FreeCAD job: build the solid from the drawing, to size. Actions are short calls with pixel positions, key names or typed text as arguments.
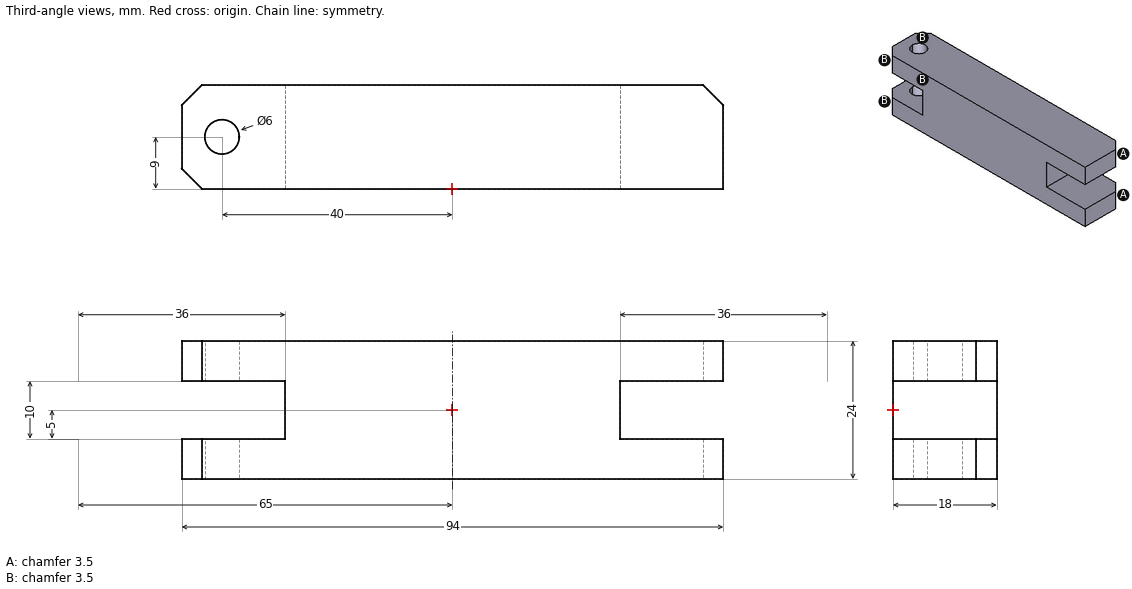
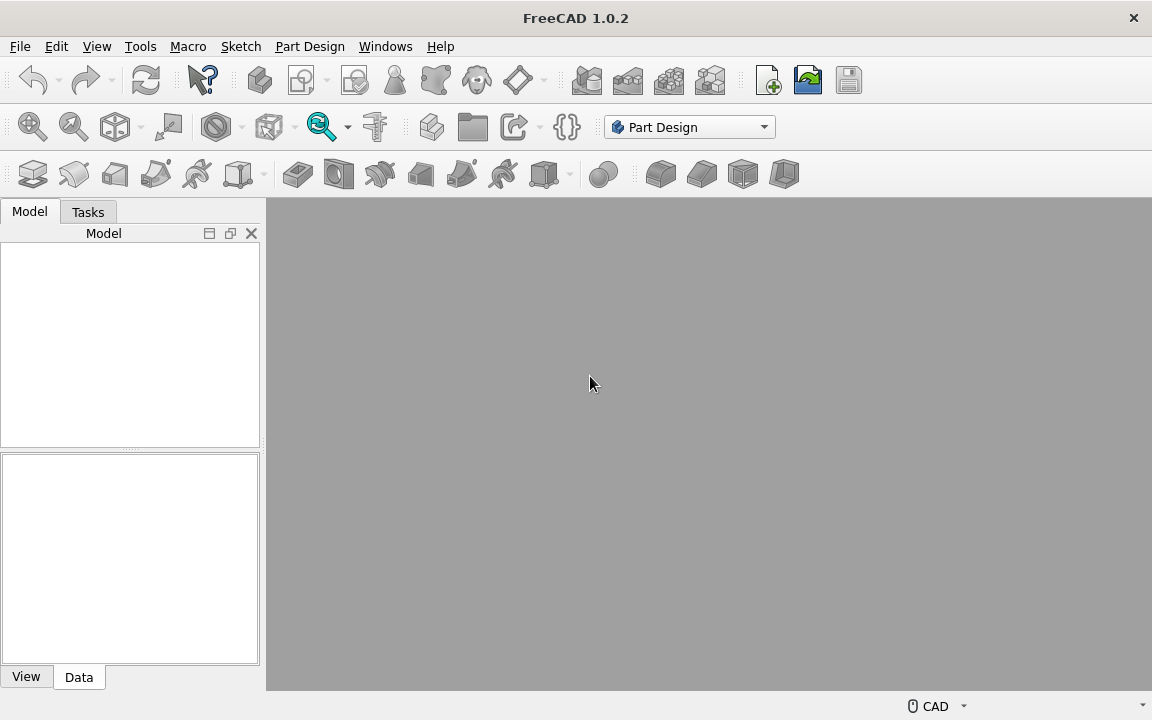
key(ctrl+n)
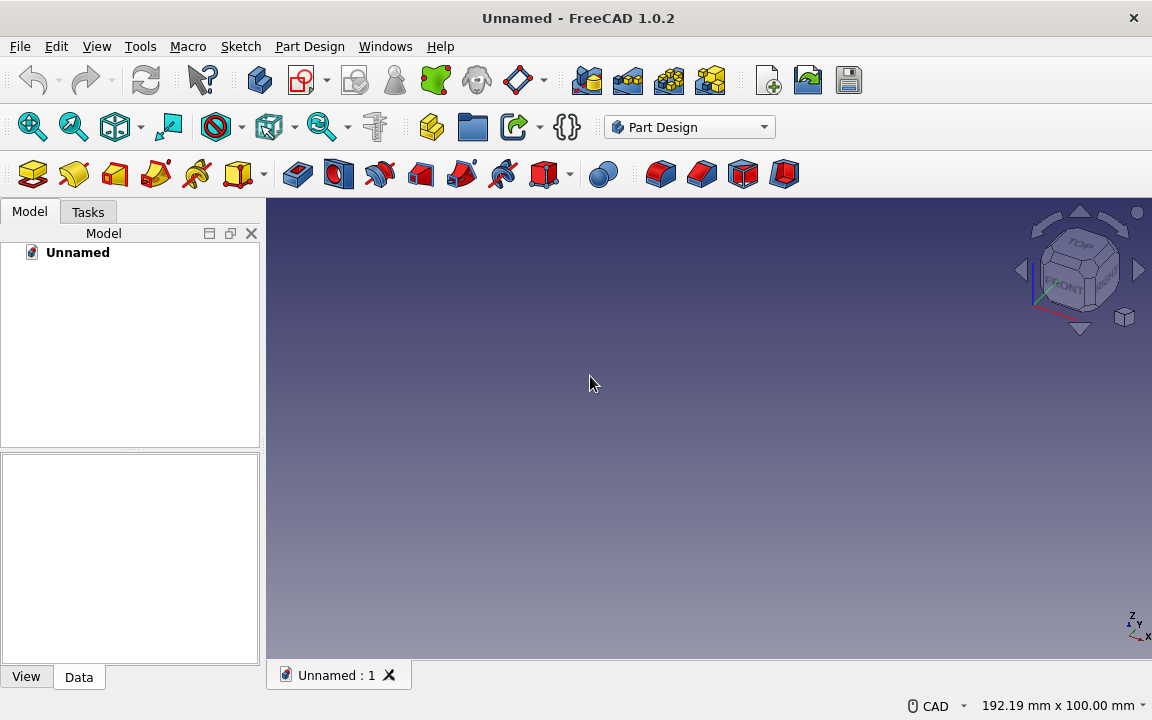
click(300, 80)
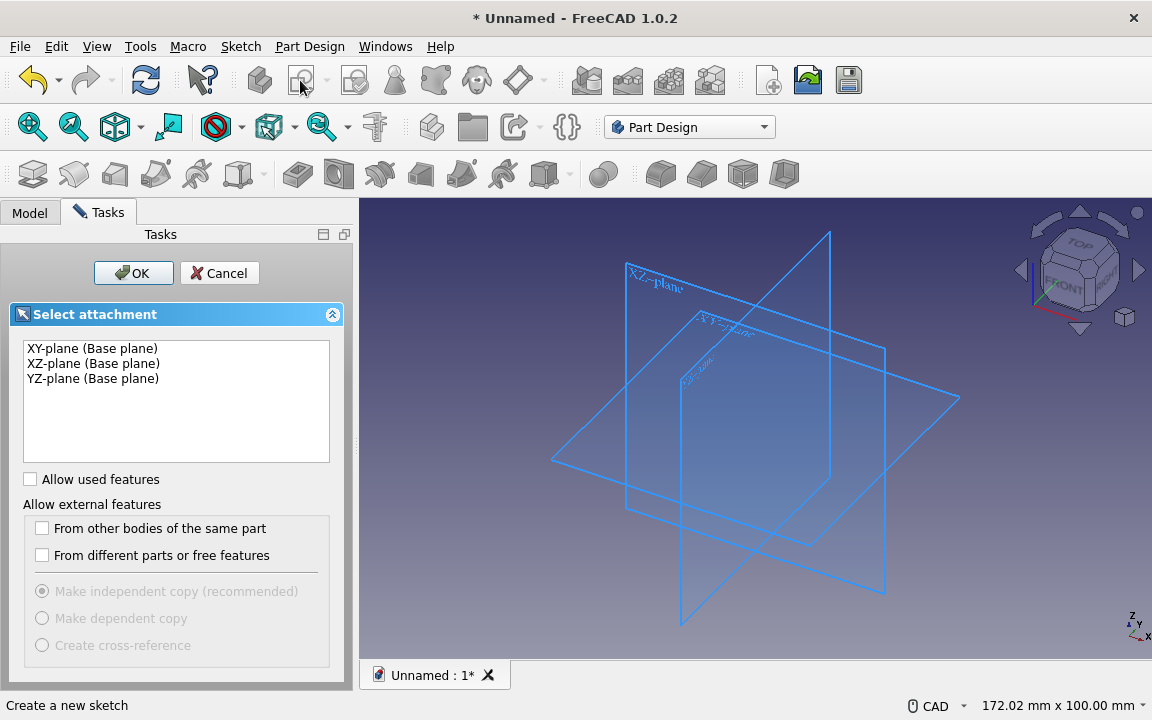
click(84, 364)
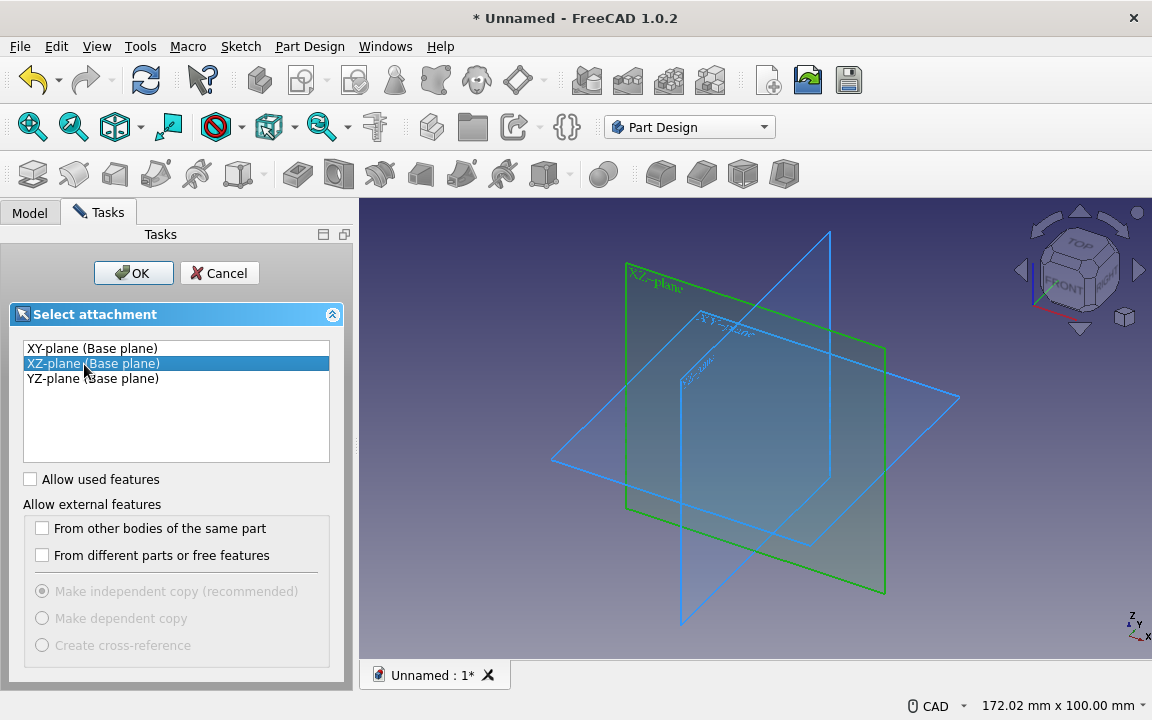
click(134, 273)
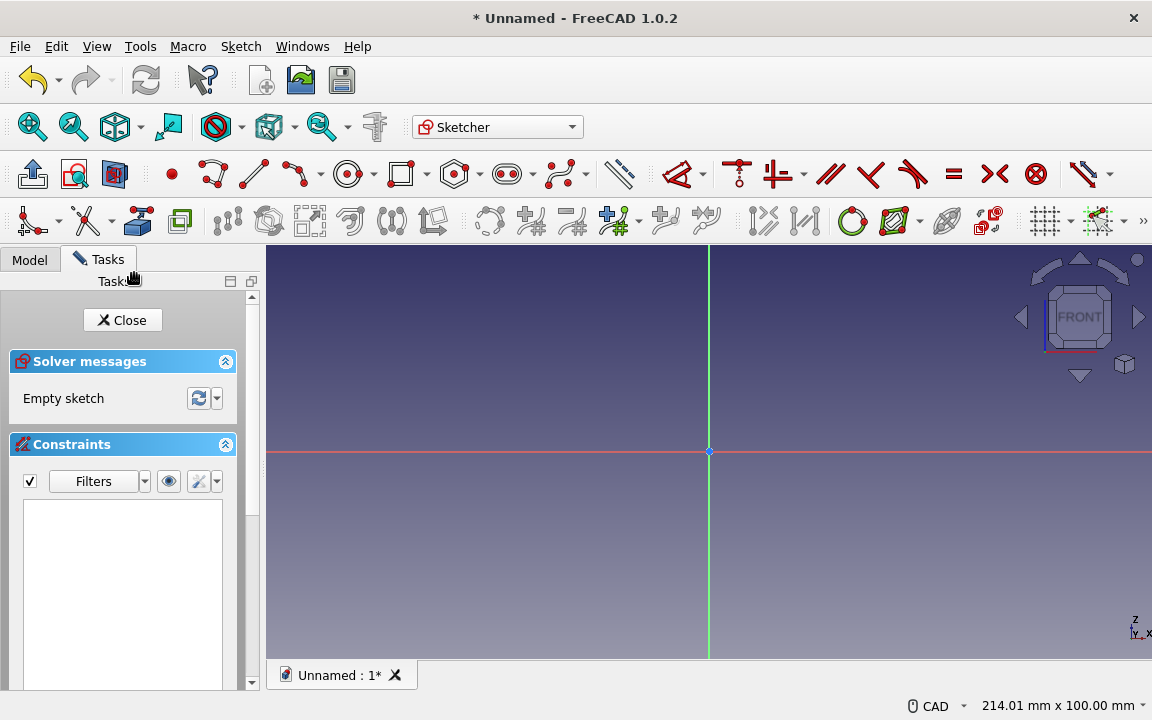
key(g)
key(v)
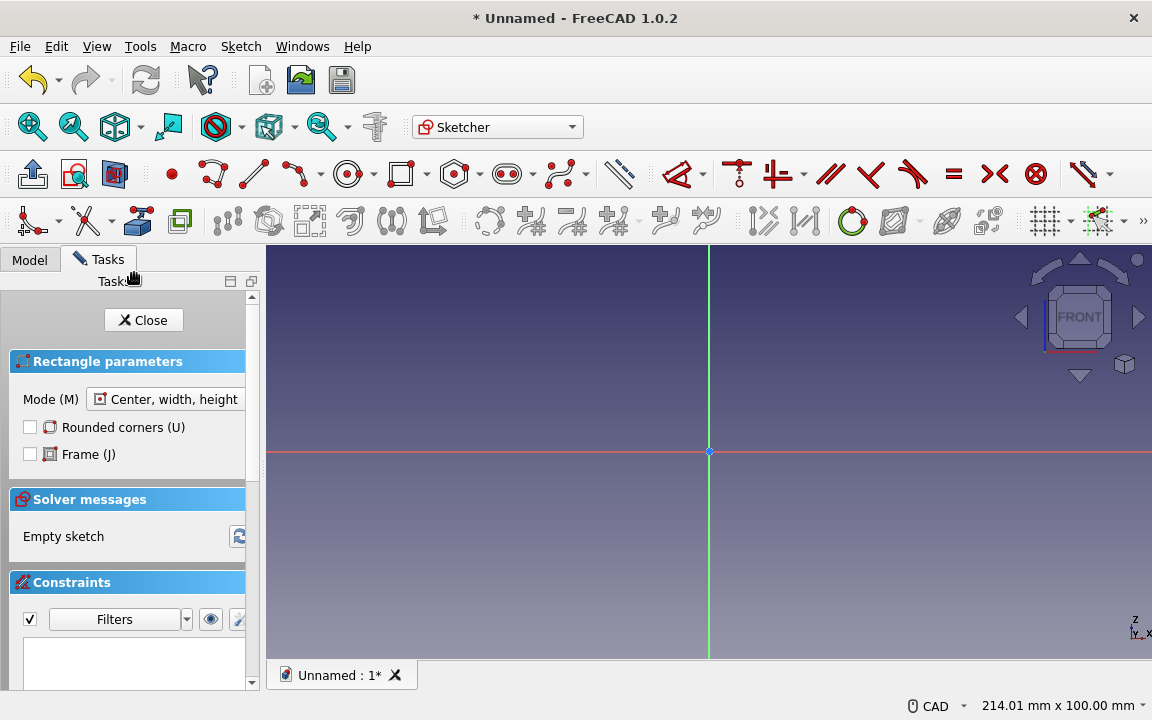
click(709, 452)
move(904, 402)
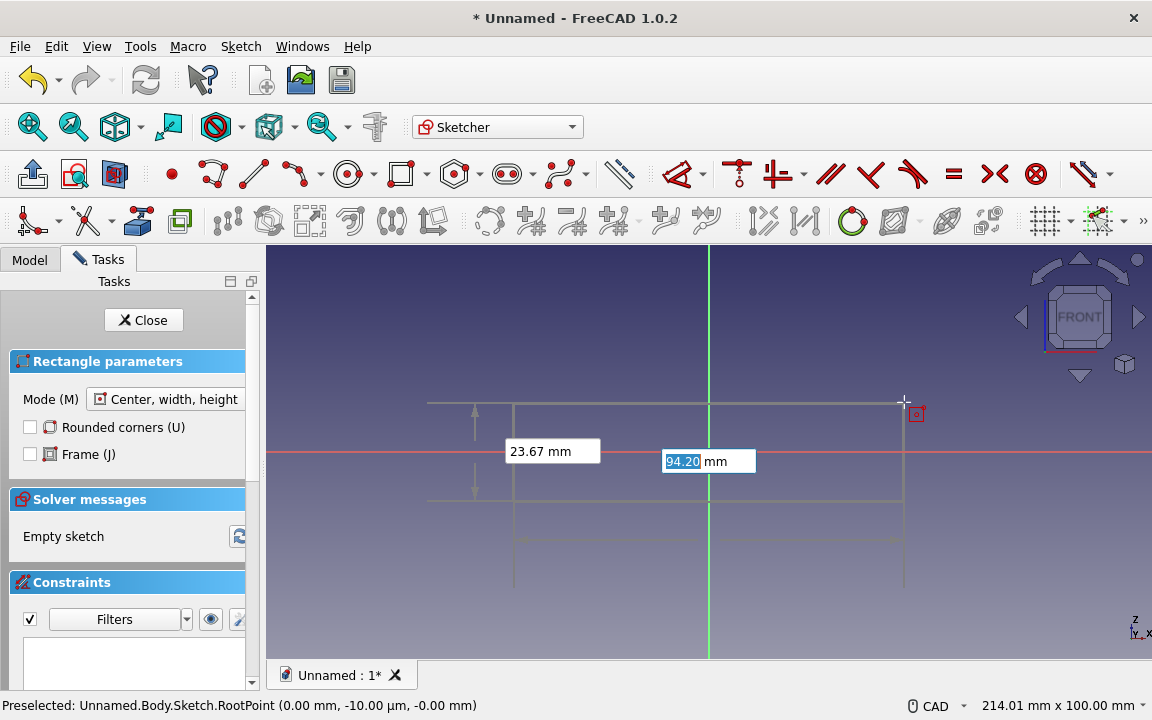
text(94)
key(Tab)
text(24)
key(Return)
key(Escape)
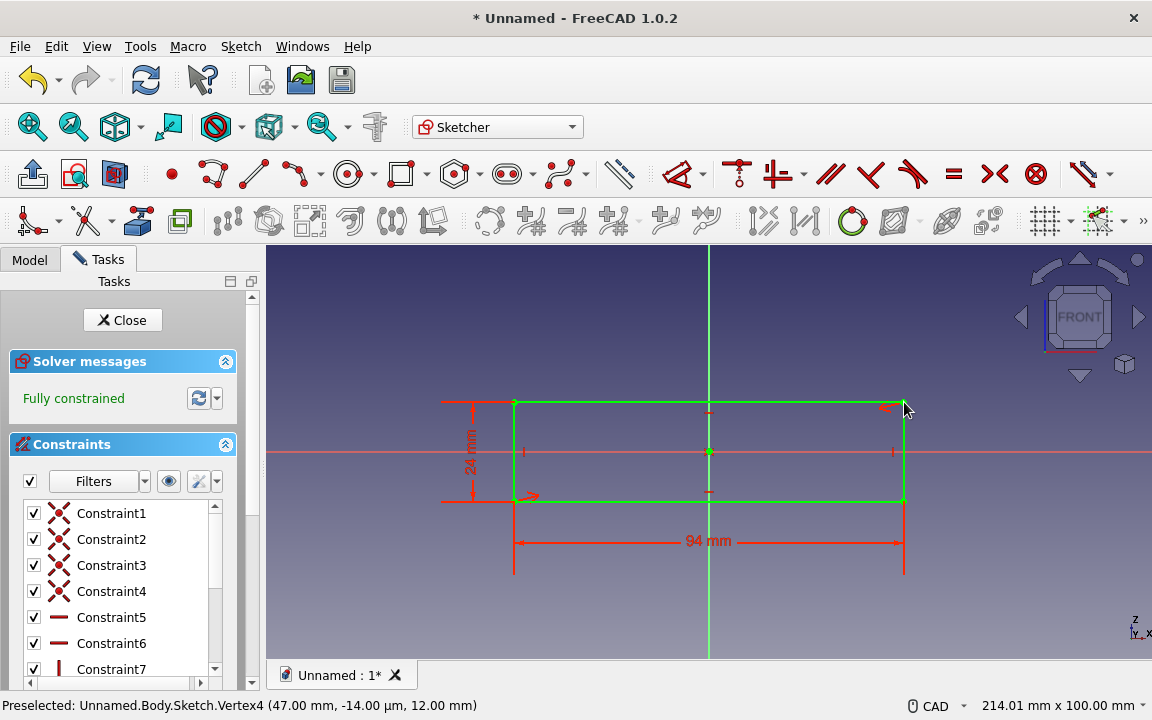
click(123, 320)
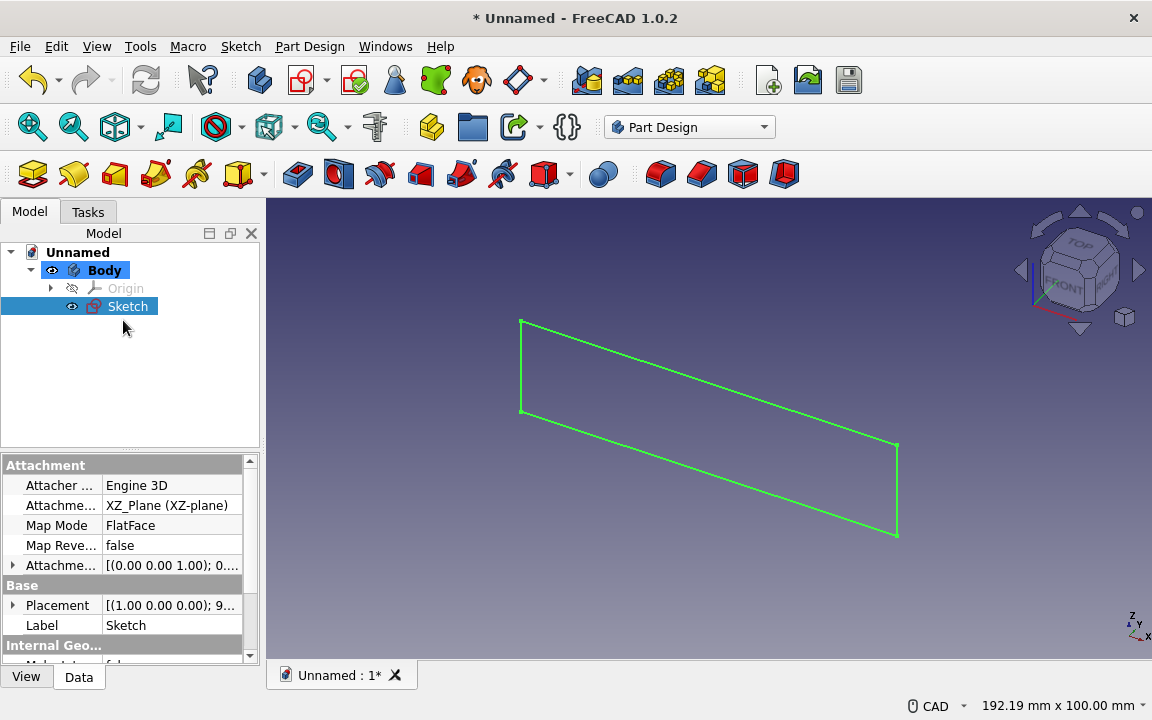
click(33, 174)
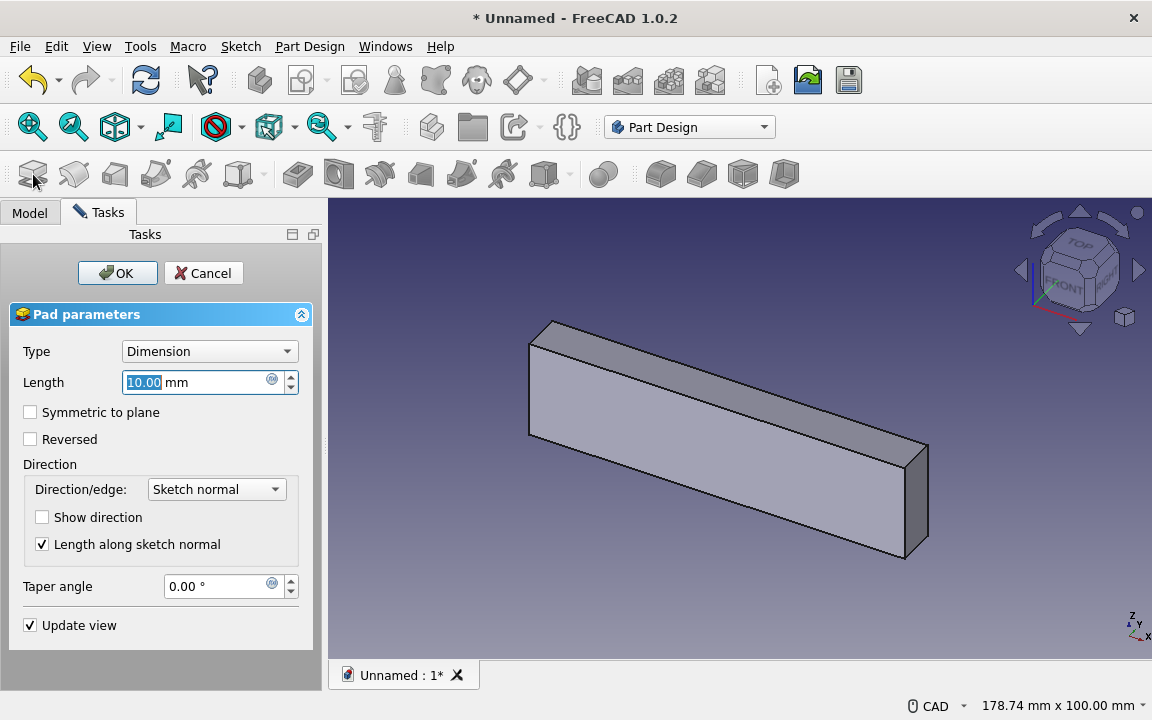
text(18)
key(Tab)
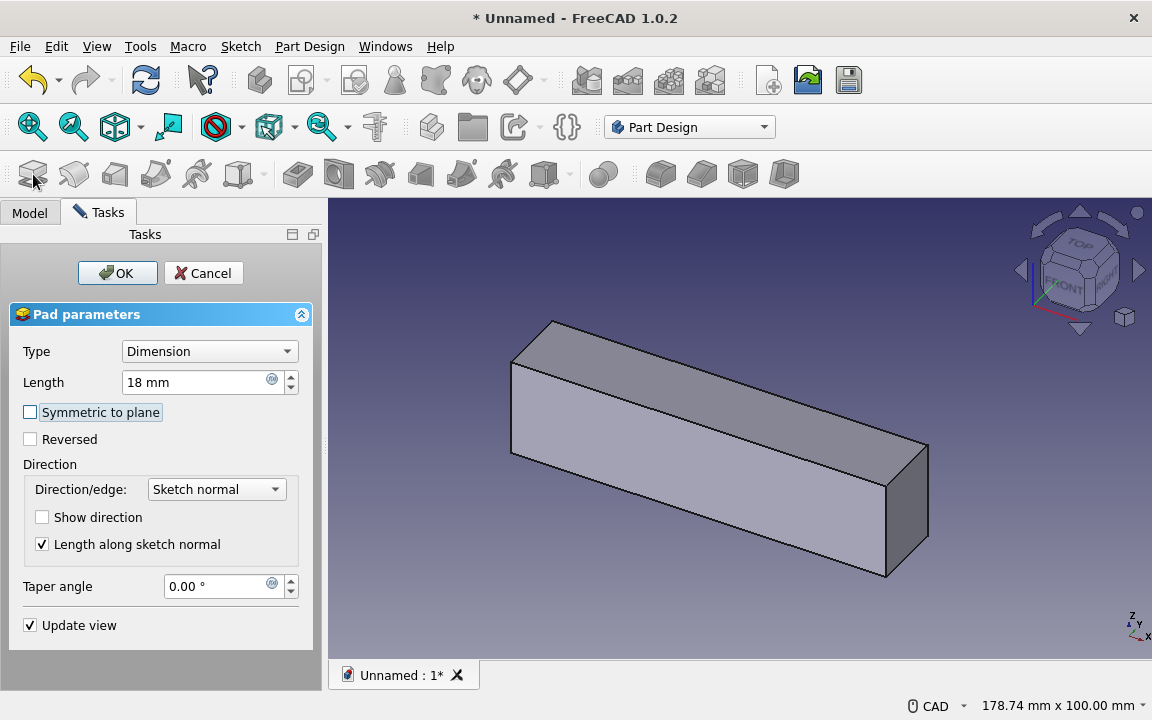
click(31, 439)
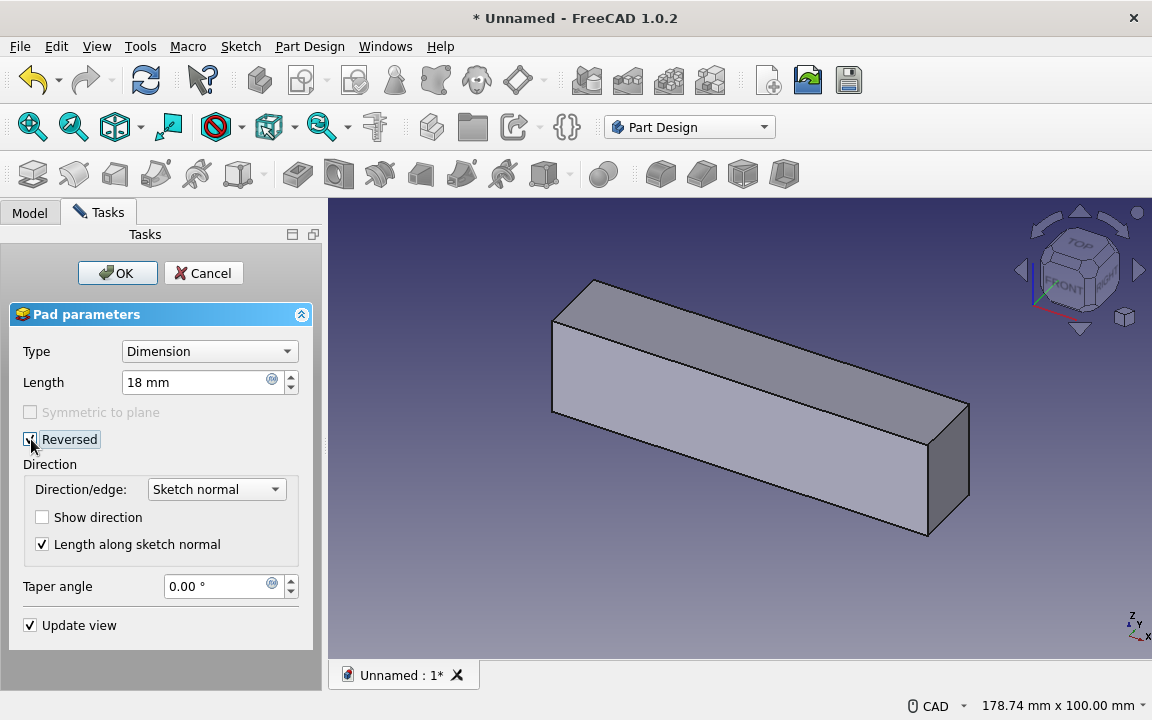
click(118, 273)